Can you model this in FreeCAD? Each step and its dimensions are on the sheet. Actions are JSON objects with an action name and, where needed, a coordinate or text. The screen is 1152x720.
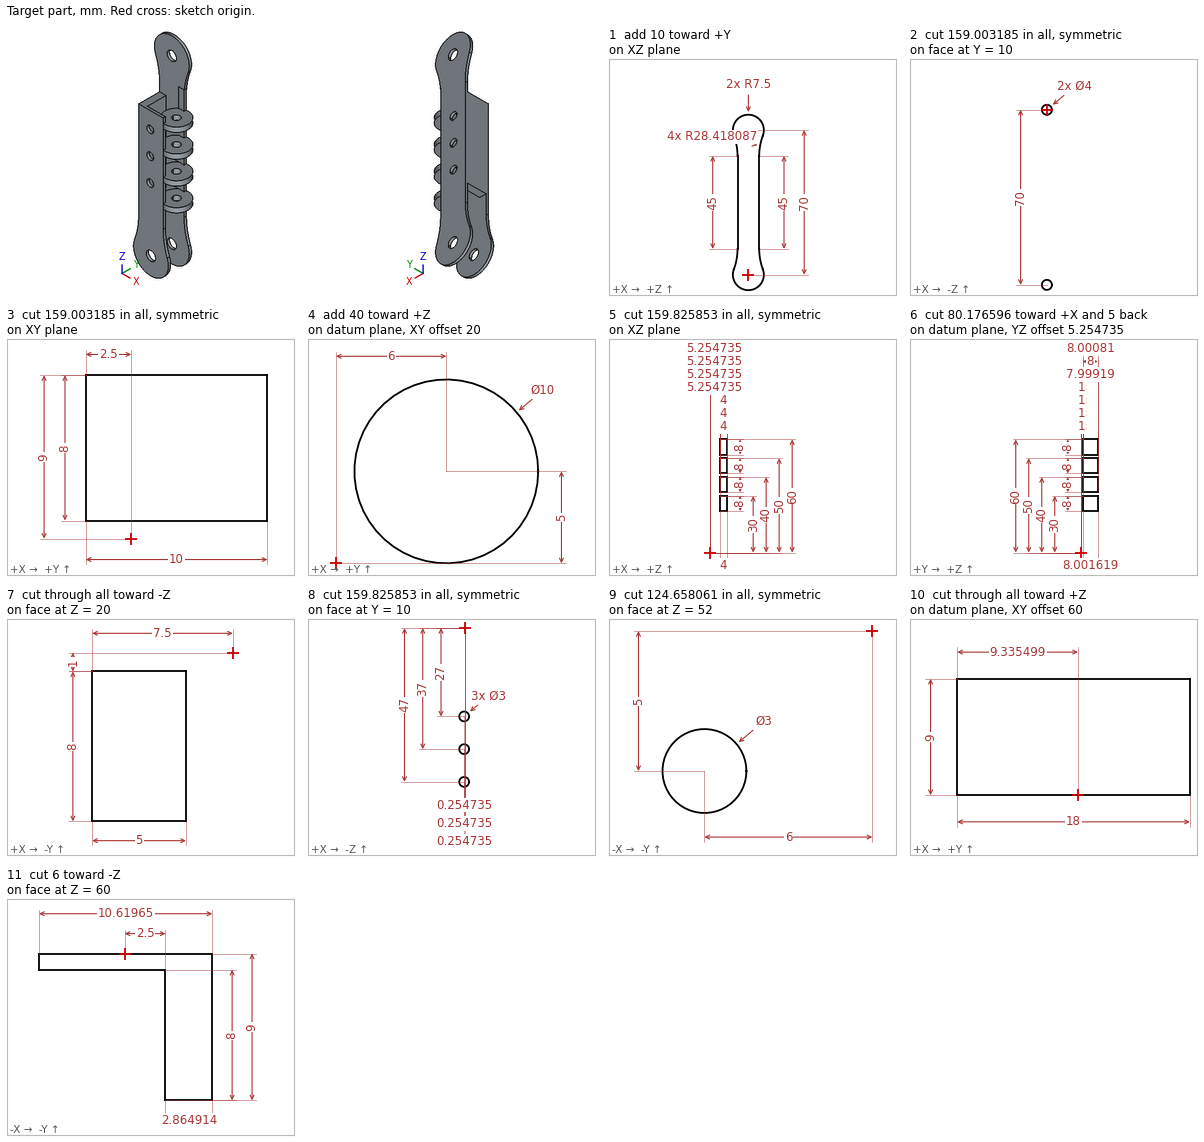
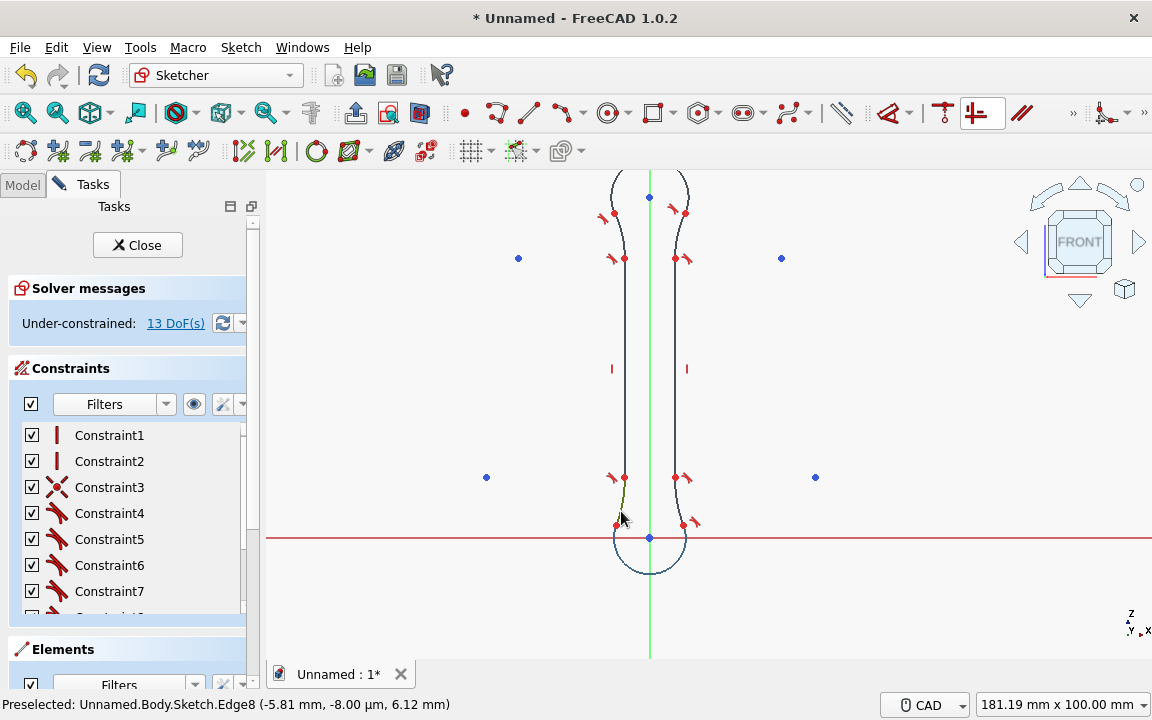
{"action": "key", "text": "t"}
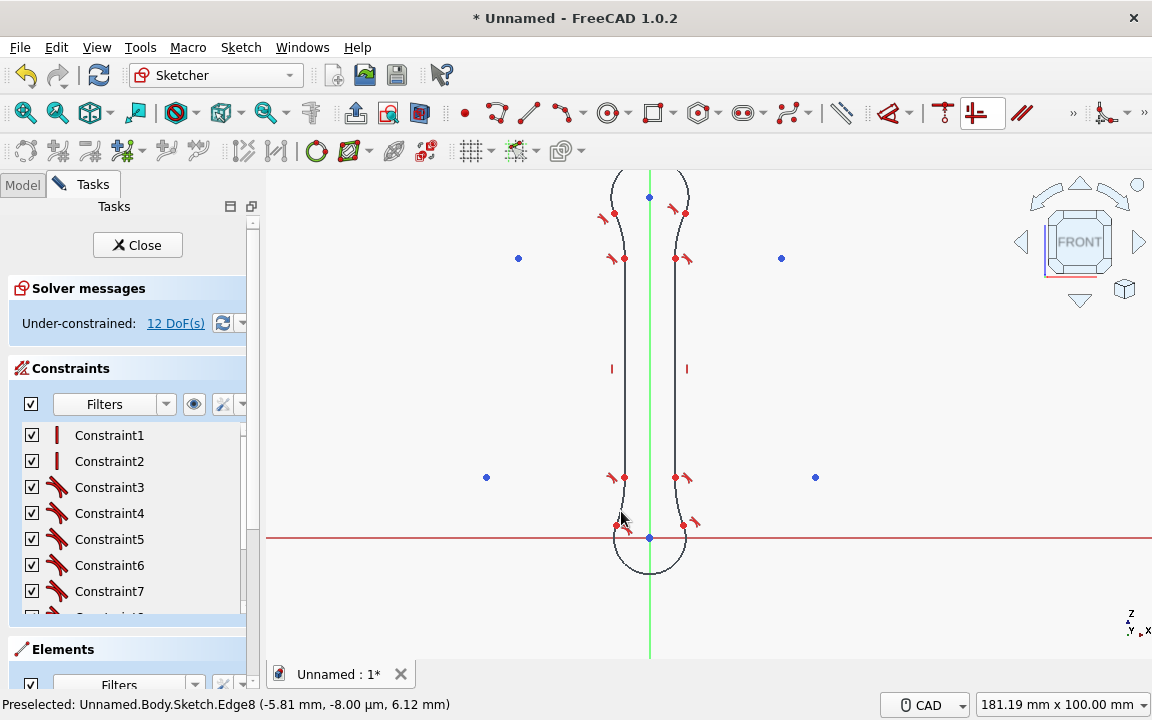
{"action": "left_click_drag", "start_coordinate": [640, 528], "coordinate": [660, 548]}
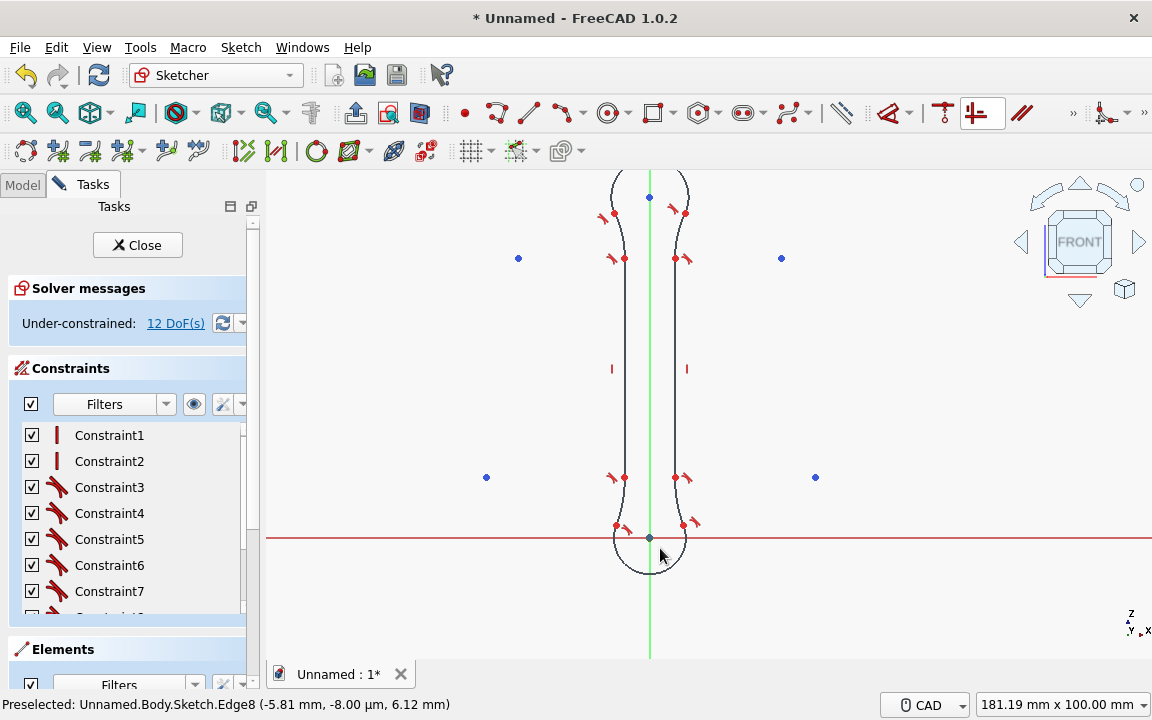
{"action": "left_click", "coordinate": [944, 114]}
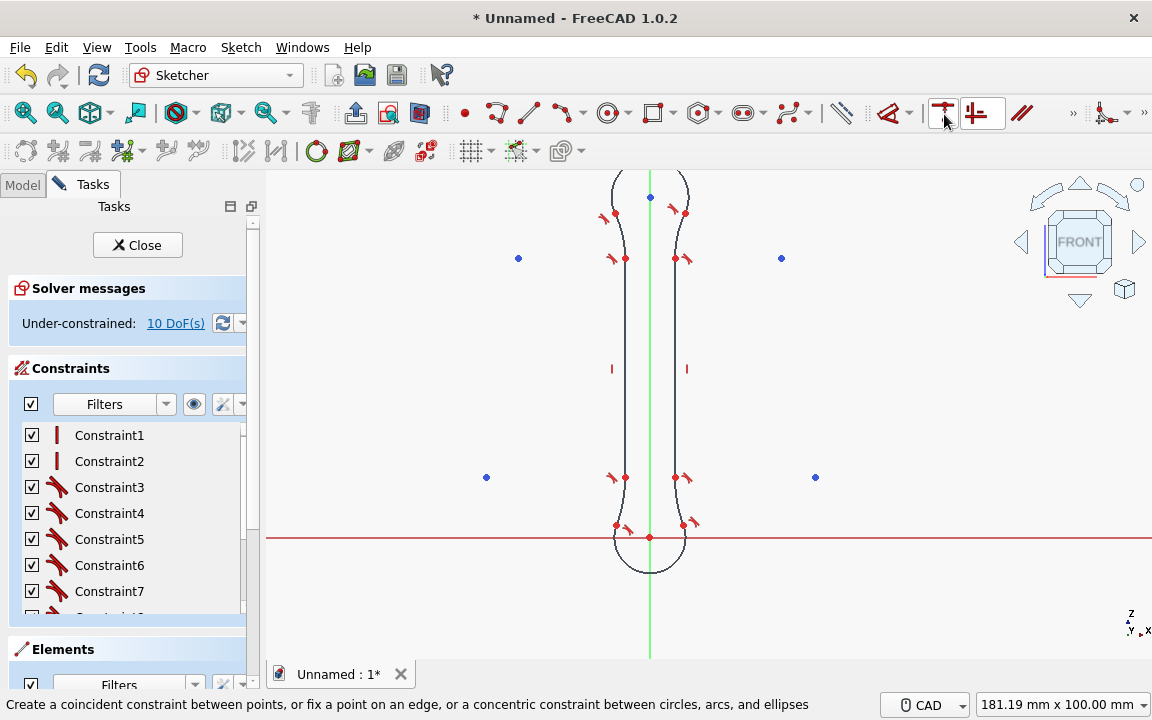
{"action": "left_click", "coordinate": [624, 244]}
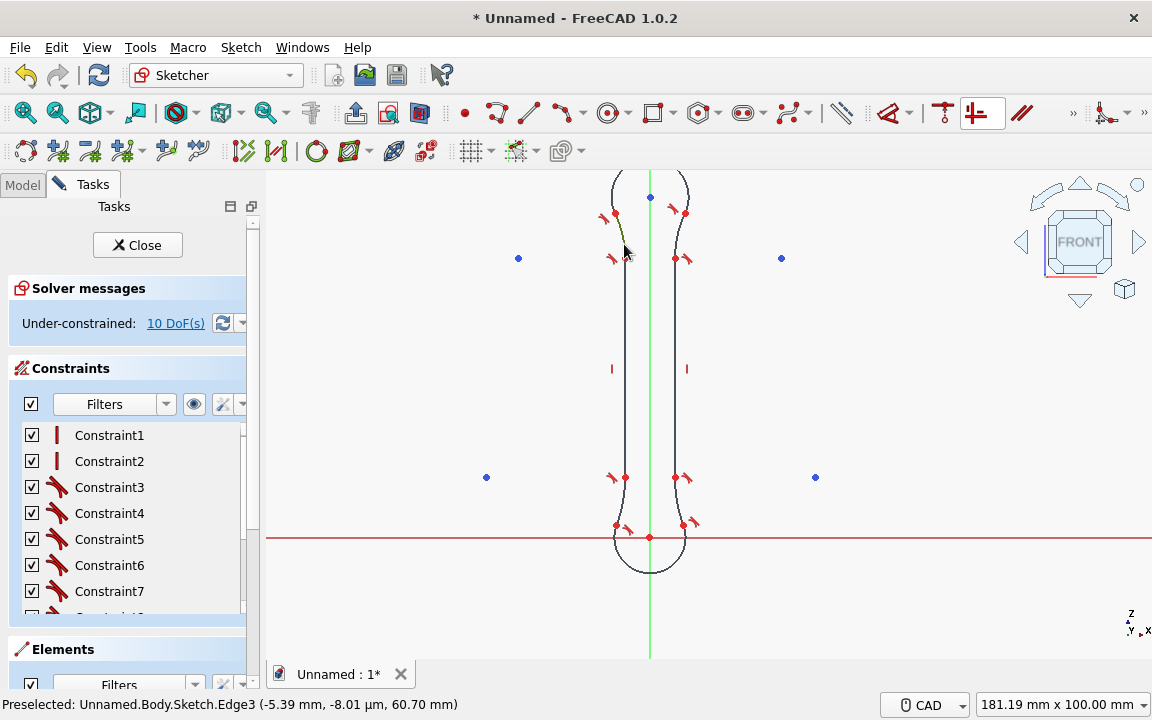
{"action": "left_click", "coordinate": [680, 226]}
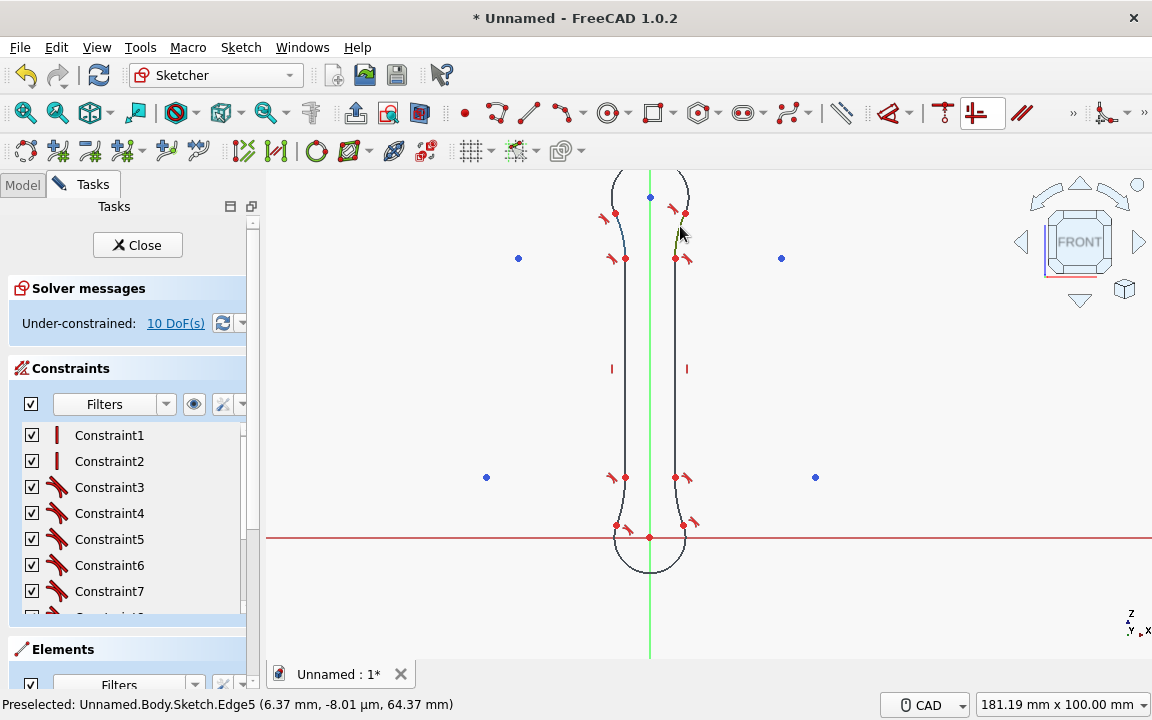
{"action": "left_click", "coordinate": [676, 492]}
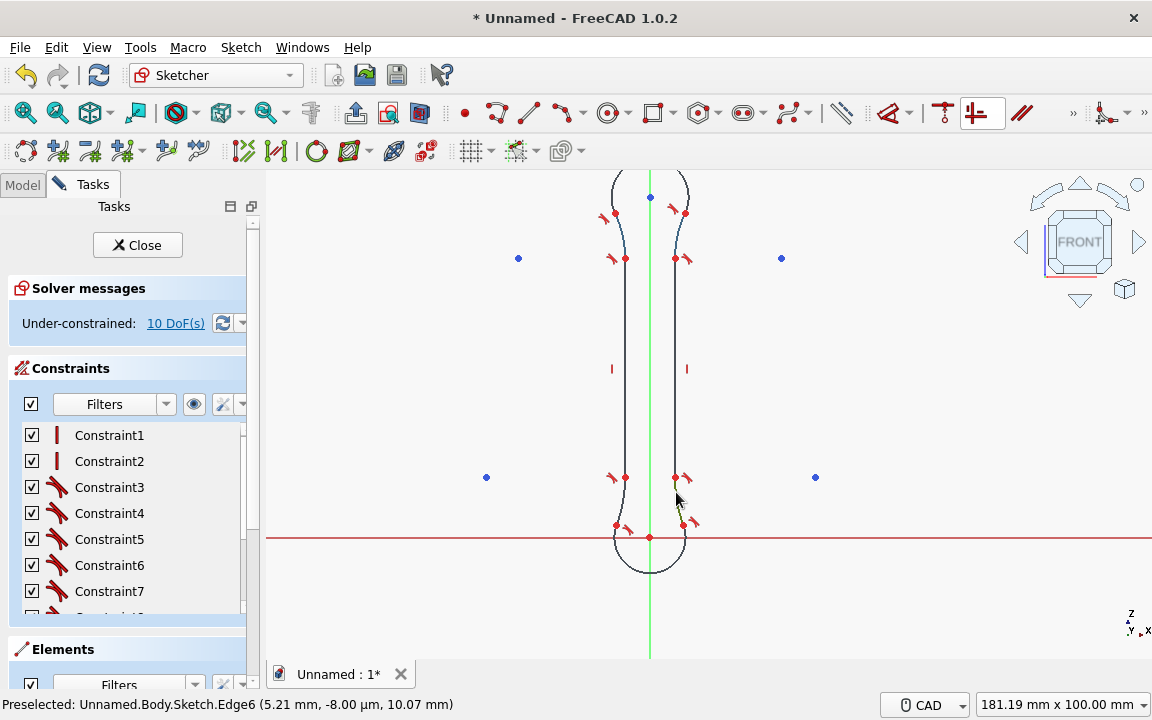
{"action": "left_click", "coordinate": [621, 511]}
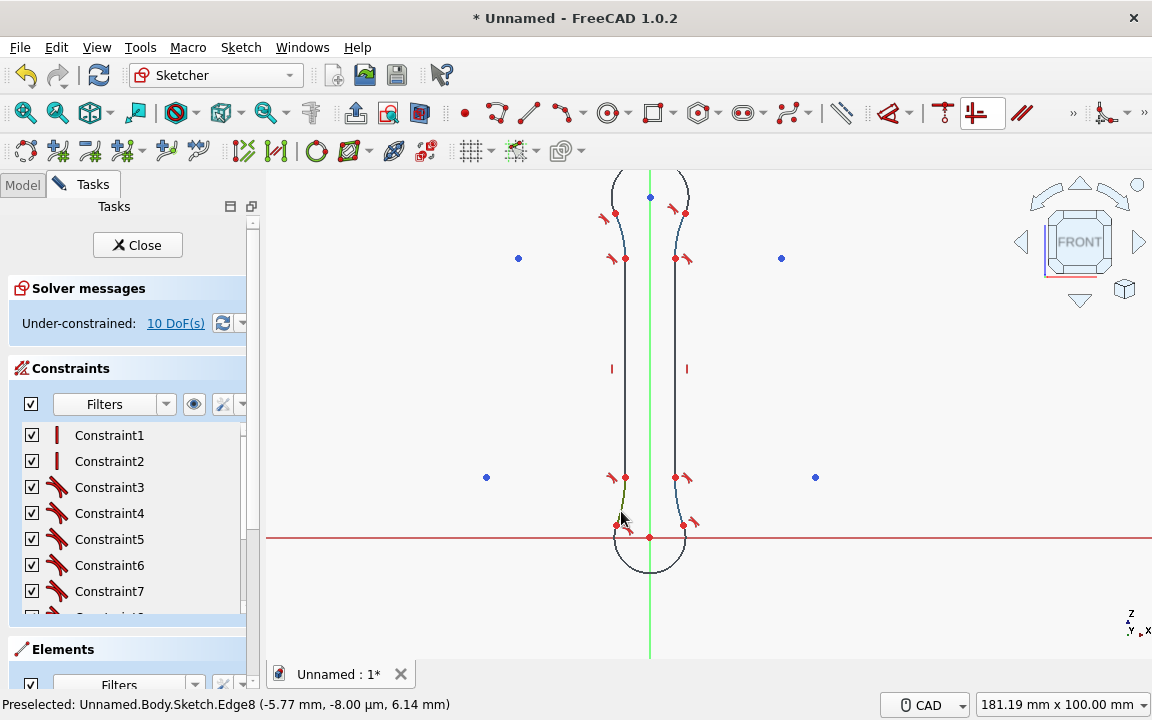
{"action": "key", "text": "e"}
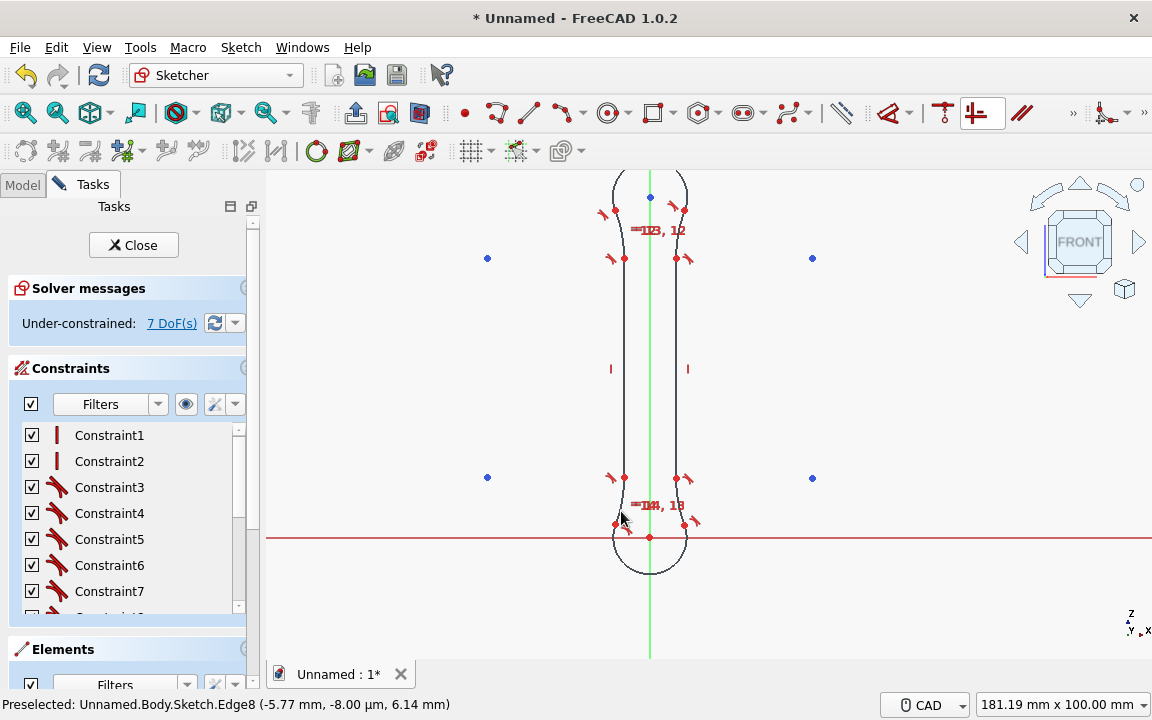
{"action": "scroll", "coordinate": [621, 512], "scroll_direction": "down", "scroll_amount": 2}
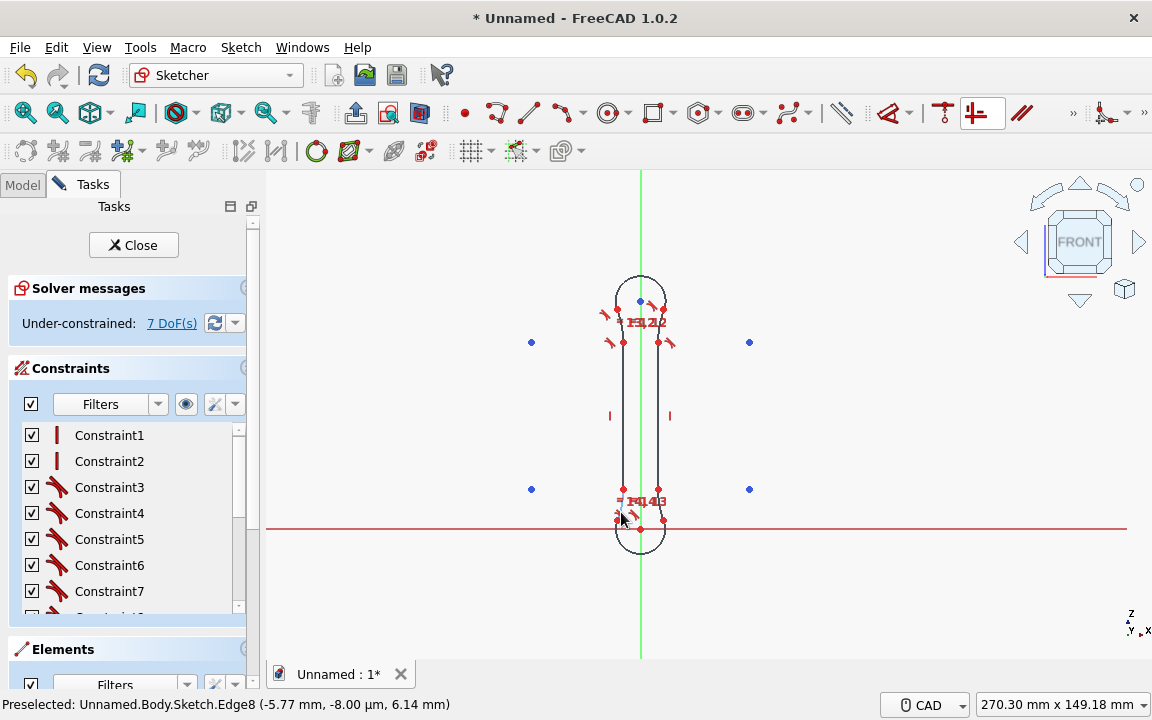
{"action": "left_click", "coordinate": [658, 283]}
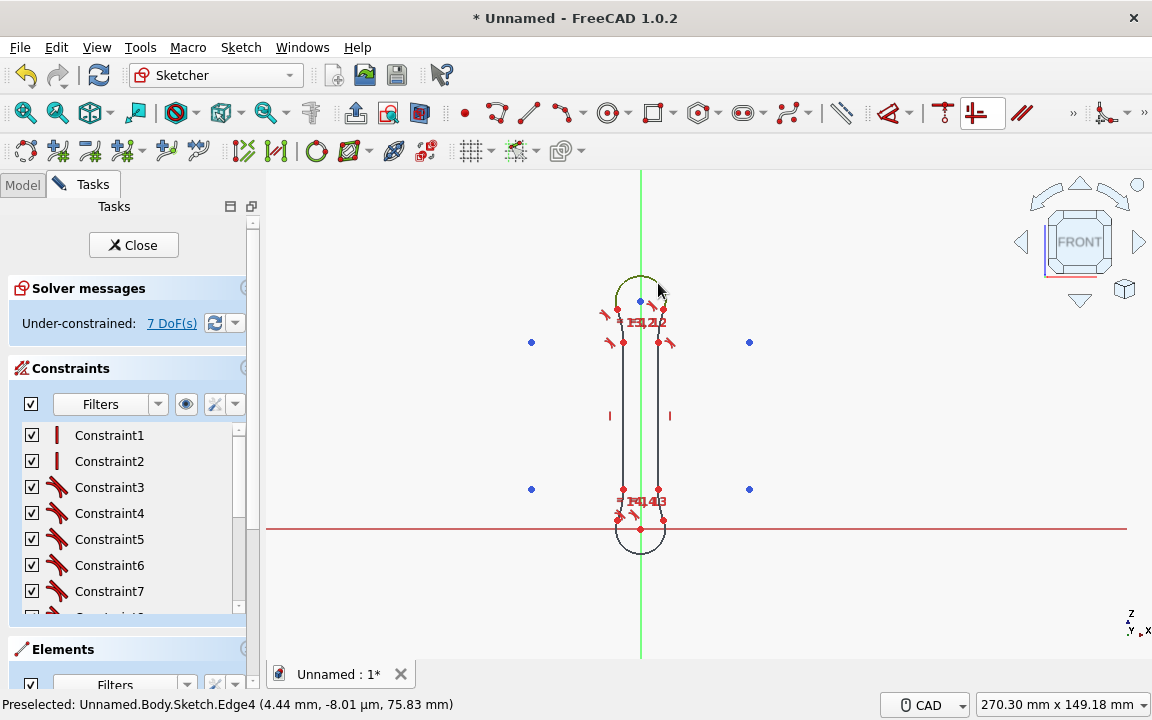
{"action": "left_click", "coordinate": [623, 547]}